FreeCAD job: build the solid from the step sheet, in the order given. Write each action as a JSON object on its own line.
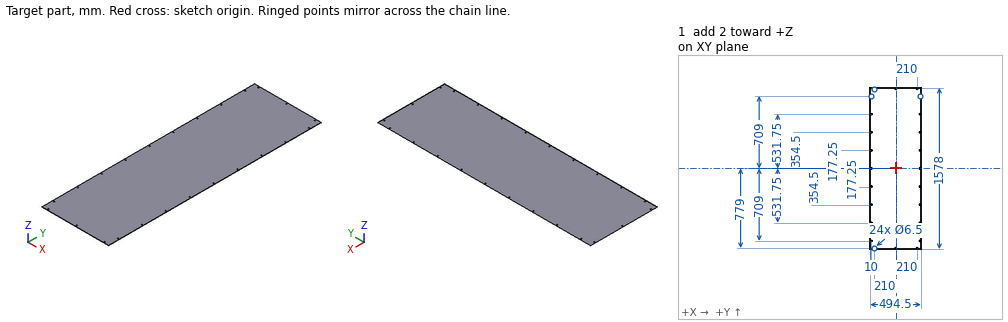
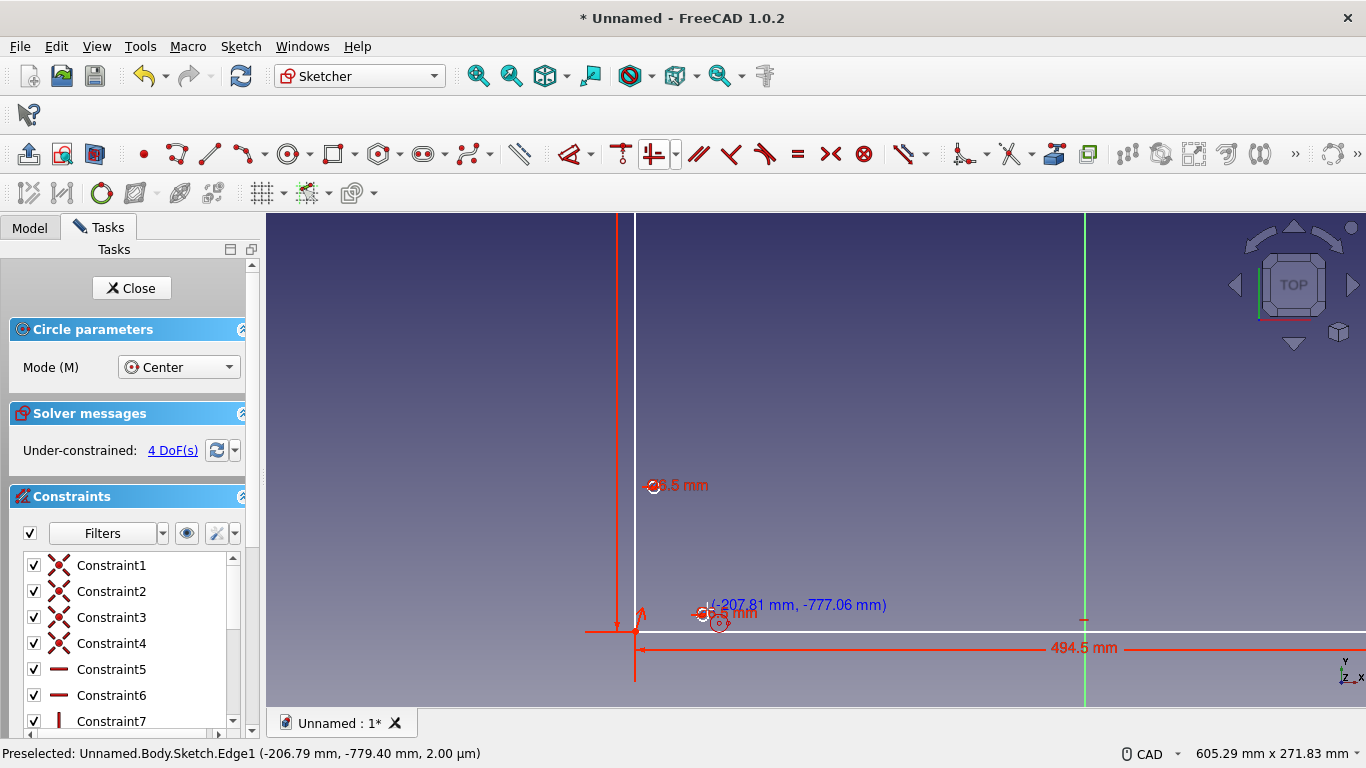
{"action": "scroll", "coordinate": [705, 617], "scroll_direction": "down", "scroll_amount": 11}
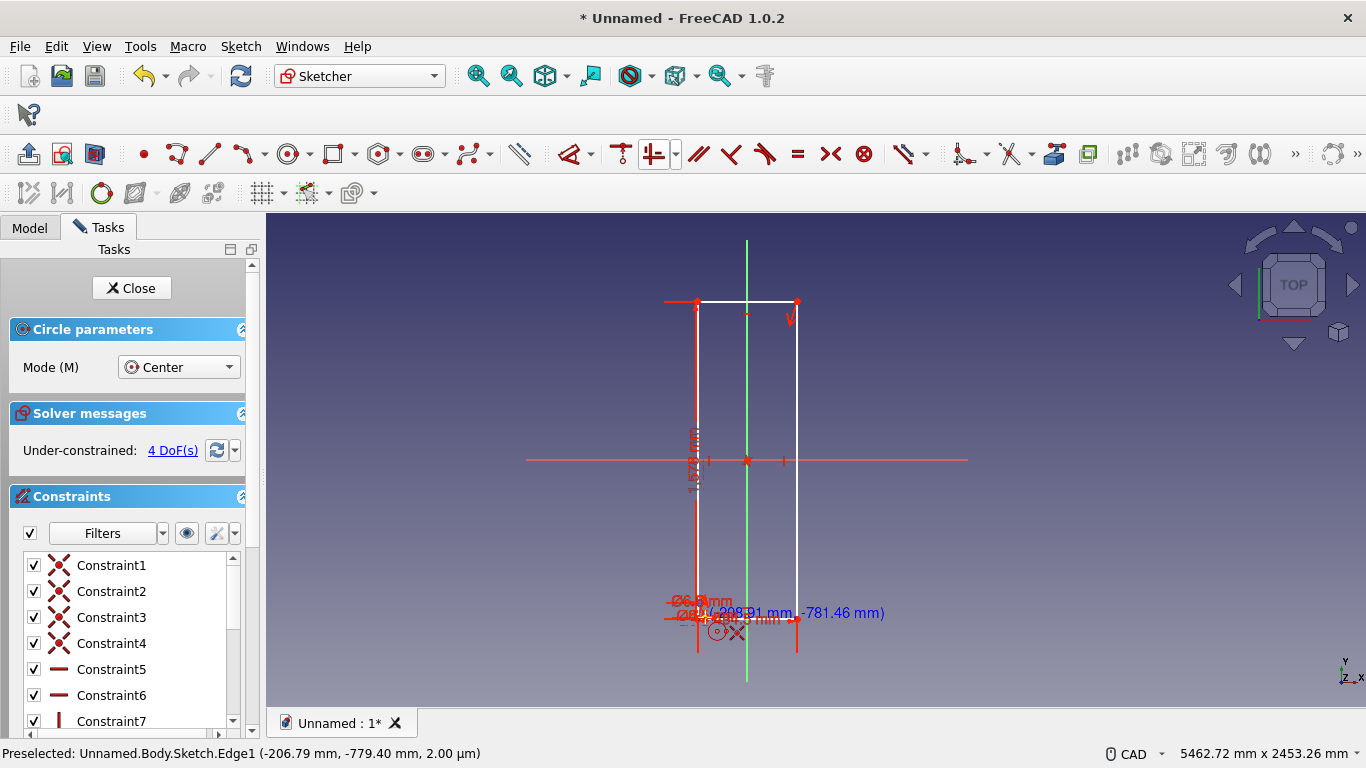
{"action": "scroll", "coordinate": [700, 568], "scroll_direction": "up", "scroll_amount": 18}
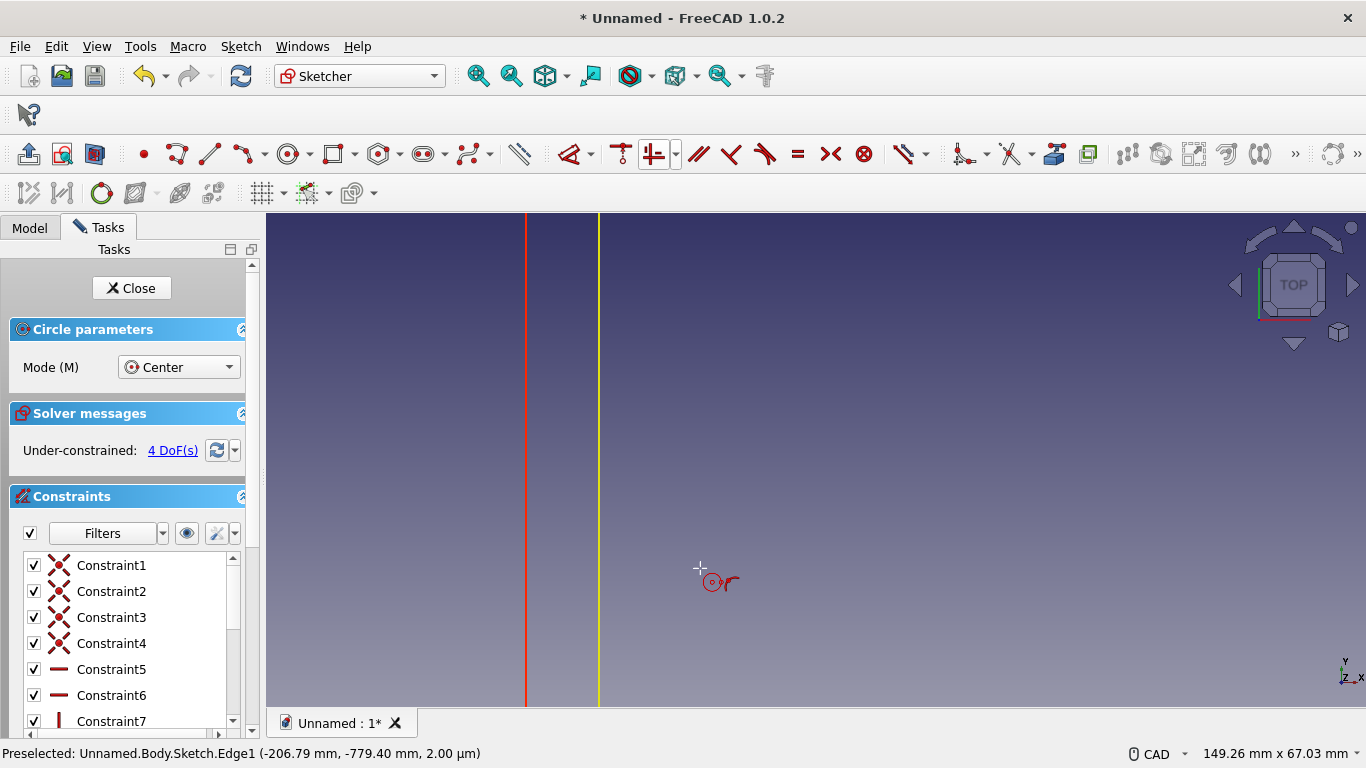
{"action": "scroll", "coordinate": [700, 568], "scroll_direction": "down", "scroll_amount": 18}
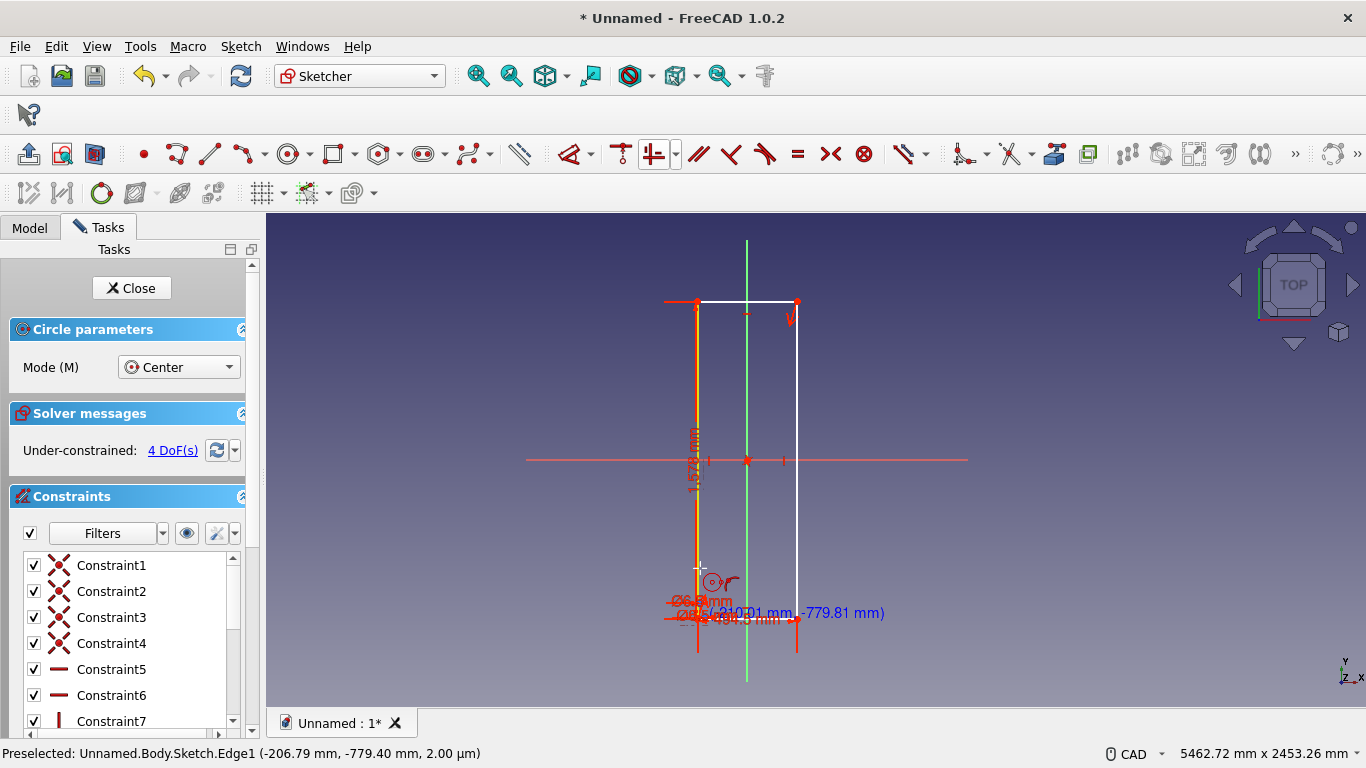
{"action": "scroll", "coordinate": [700, 568], "scroll_direction": "up", "scroll_amount": 11}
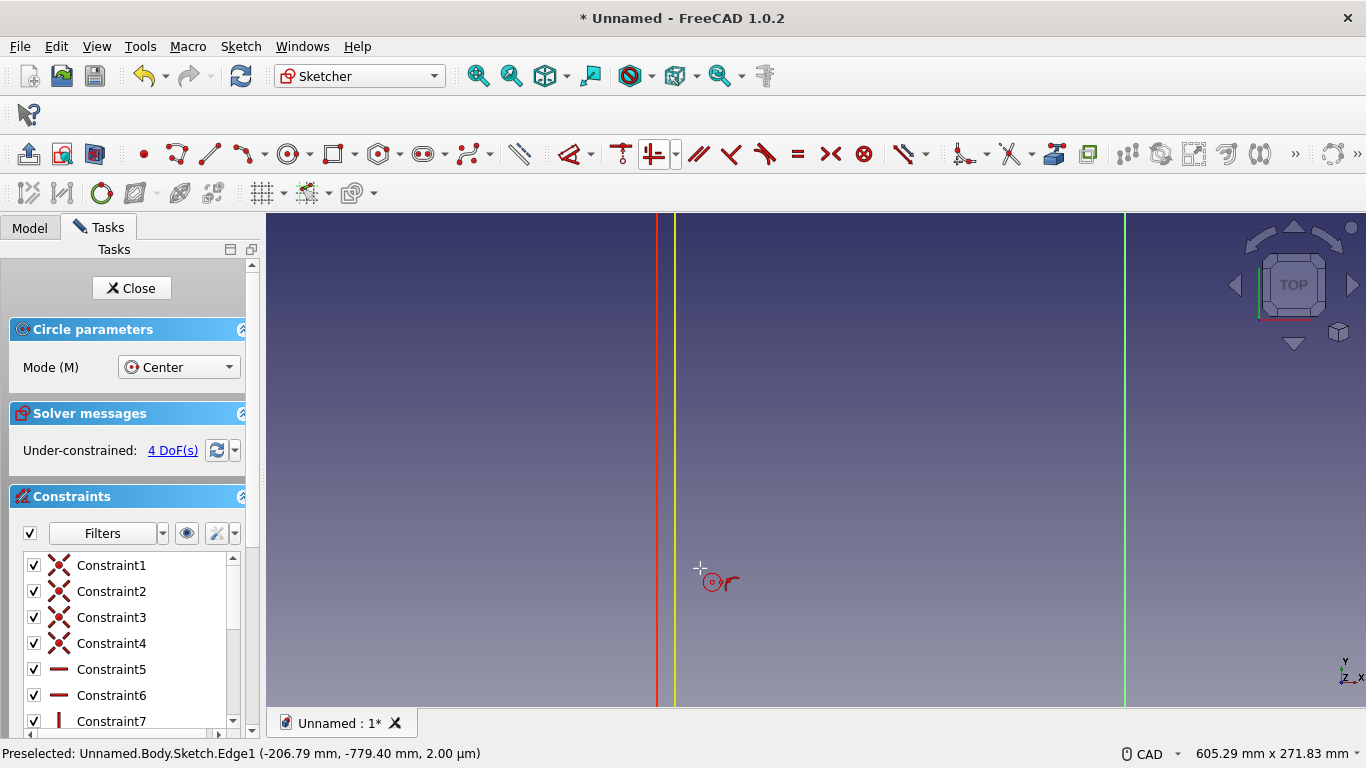
{"action": "left_click", "coordinate": [694, 558]}
{"action": "mouse_move", "coordinate": [698, 554]}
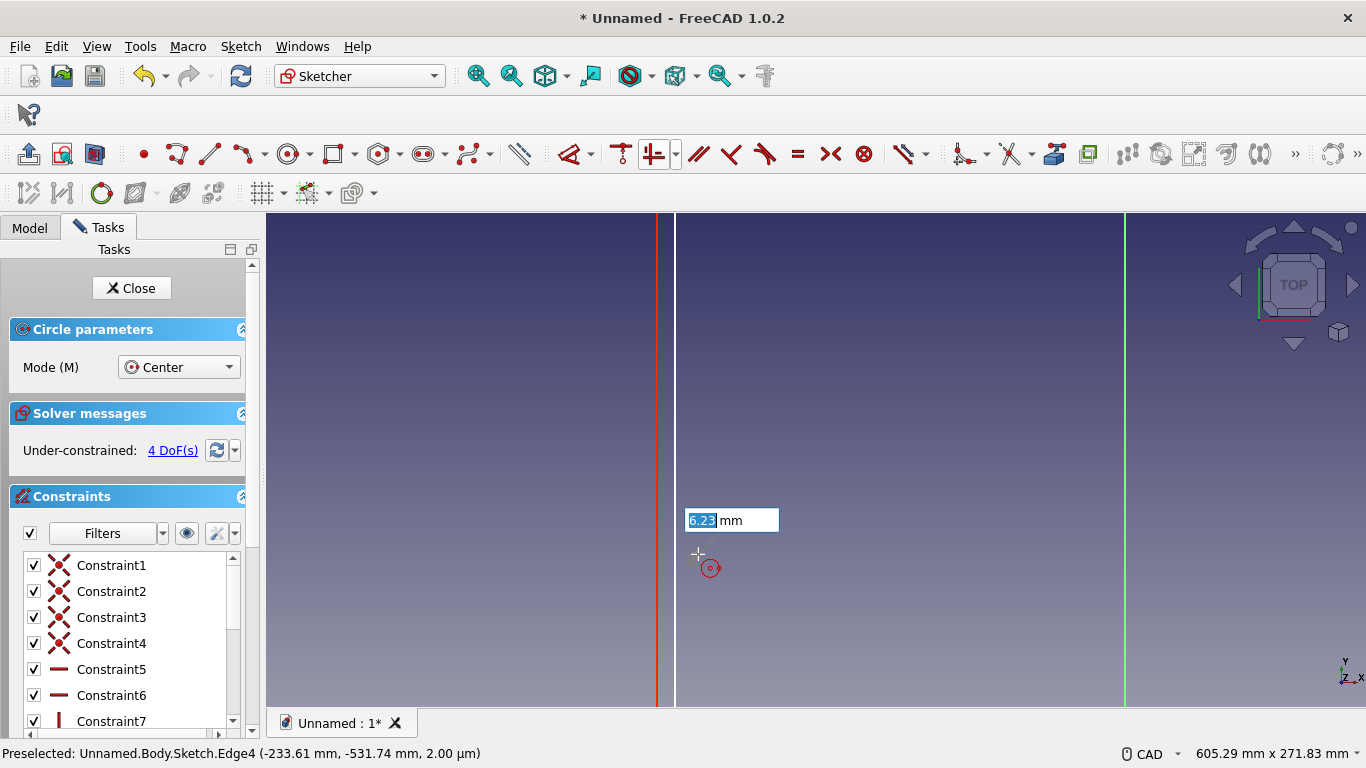
{"action": "type", "text": "6.5"}
{"action": "key", "text": "Return"}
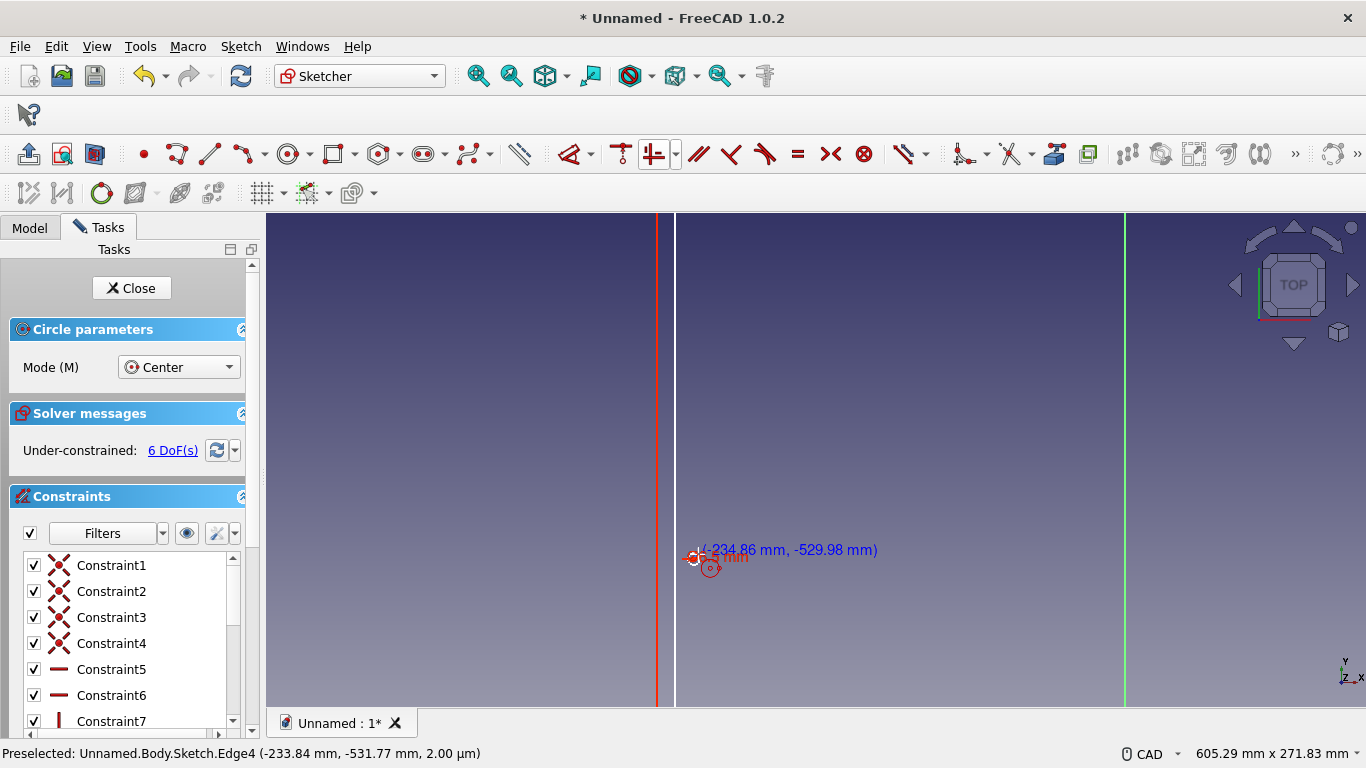
{"action": "scroll", "coordinate": [700, 568], "scroll_direction": "down", "scroll_amount": 11}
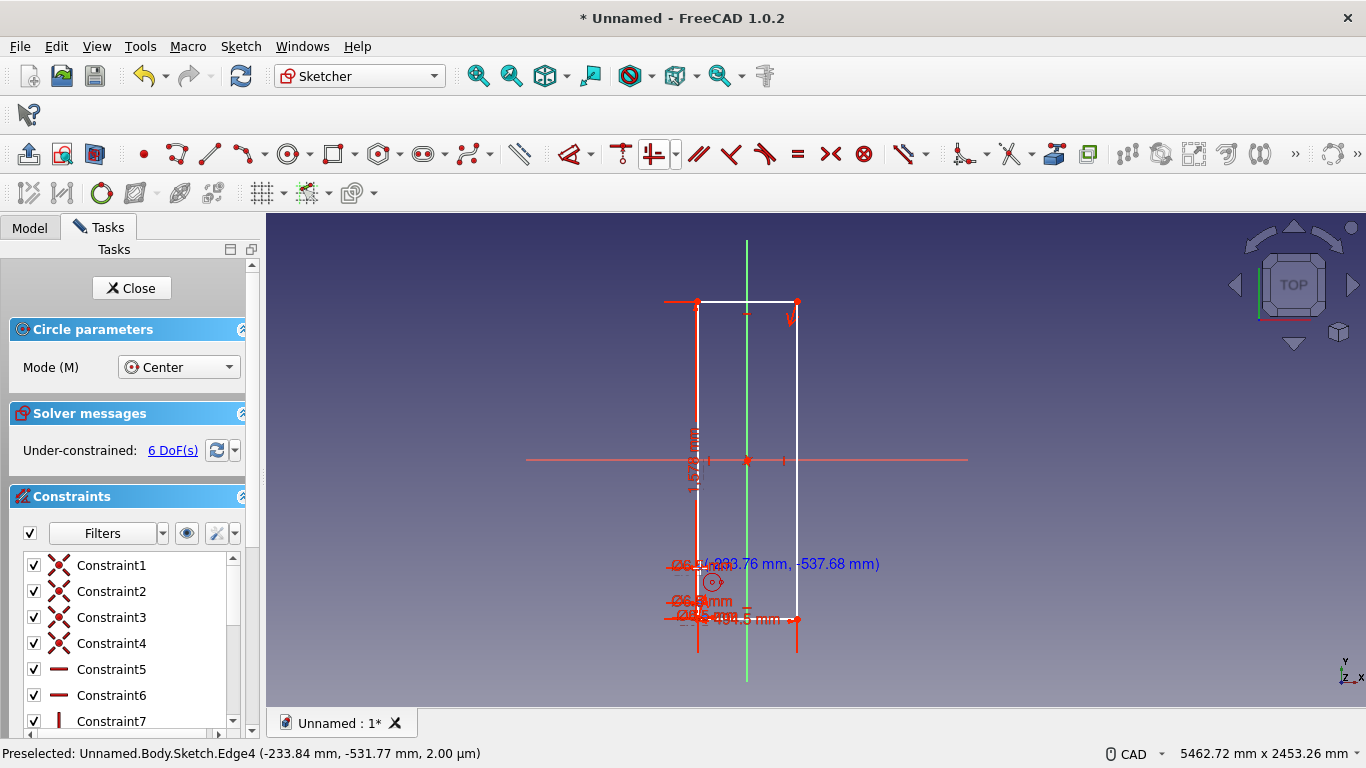
{"action": "scroll", "coordinate": [700, 532], "scroll_direction": "up", "scroll_amount": 18}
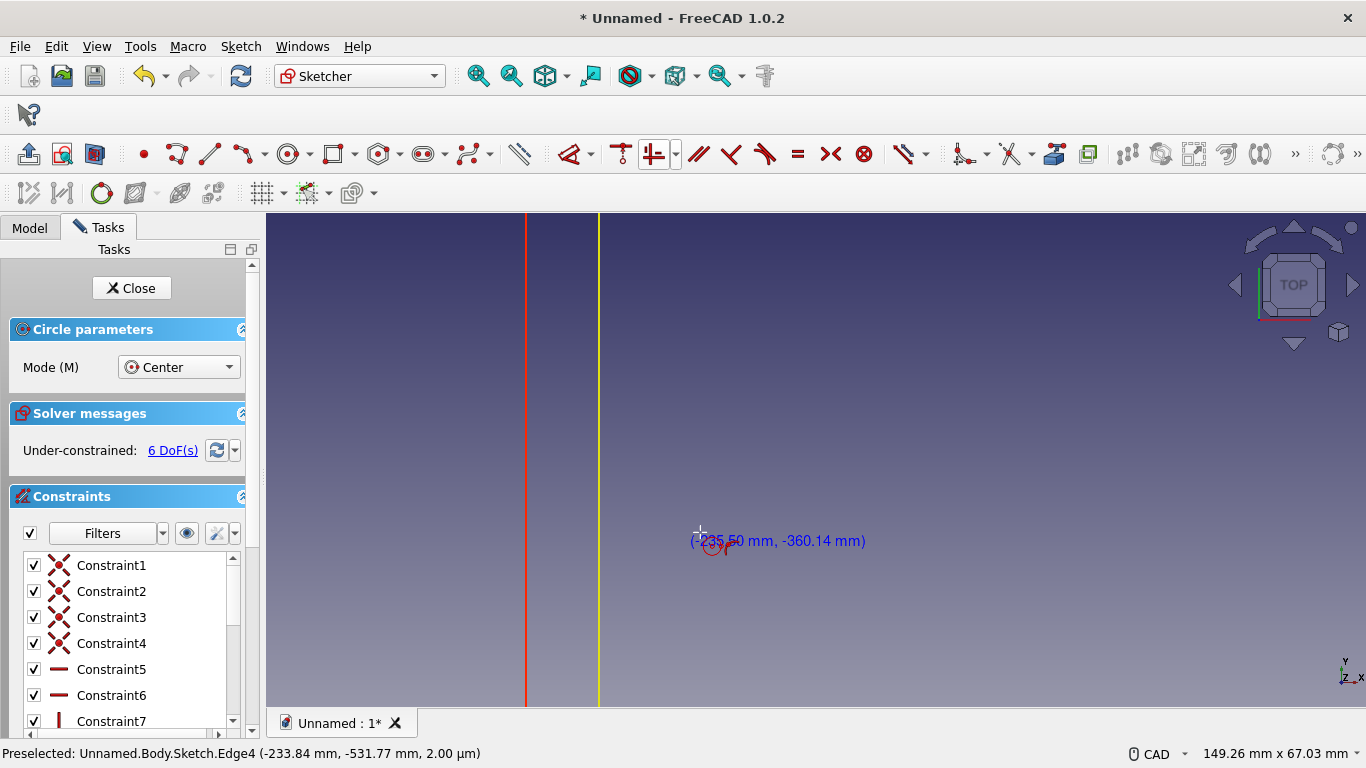
{"action": "scroll", "coordinate": [700, 532], "scroll_direction": "down", "scroll_amount": 18}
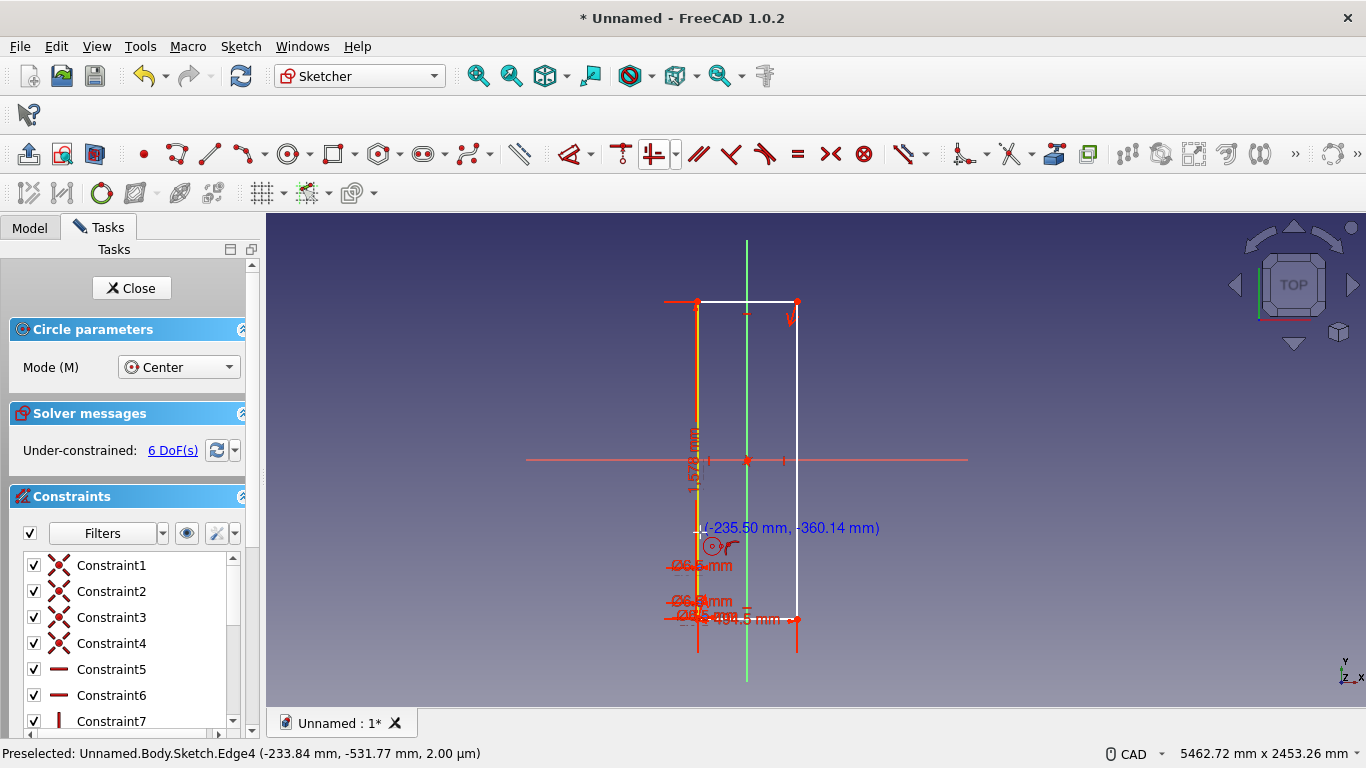
{"action": "scroll", "coordinate": [700, 532], "scroll_direction": "up", "scroll_amount": 11}